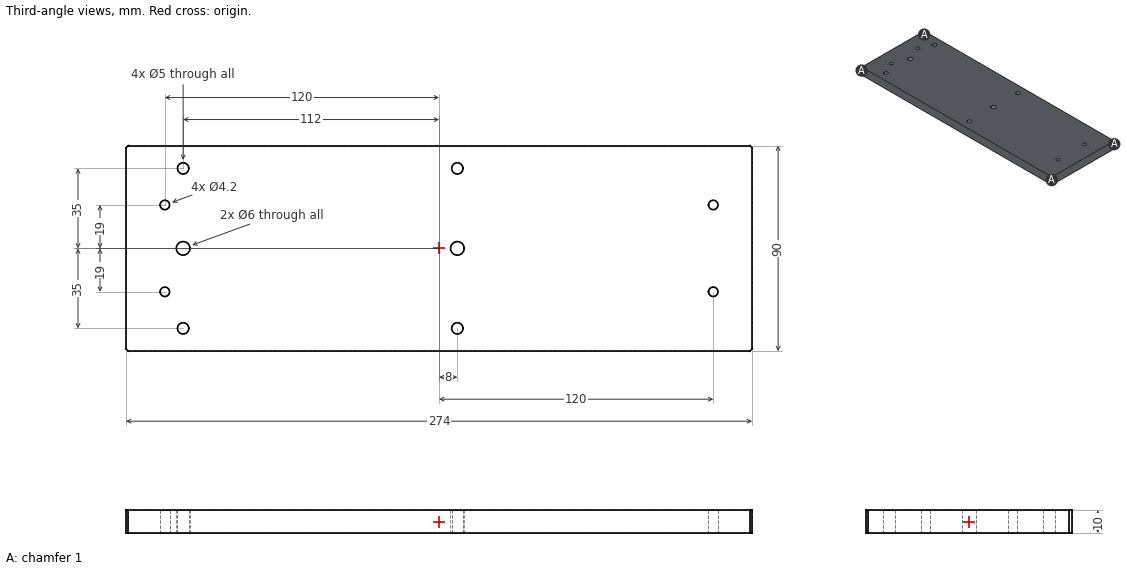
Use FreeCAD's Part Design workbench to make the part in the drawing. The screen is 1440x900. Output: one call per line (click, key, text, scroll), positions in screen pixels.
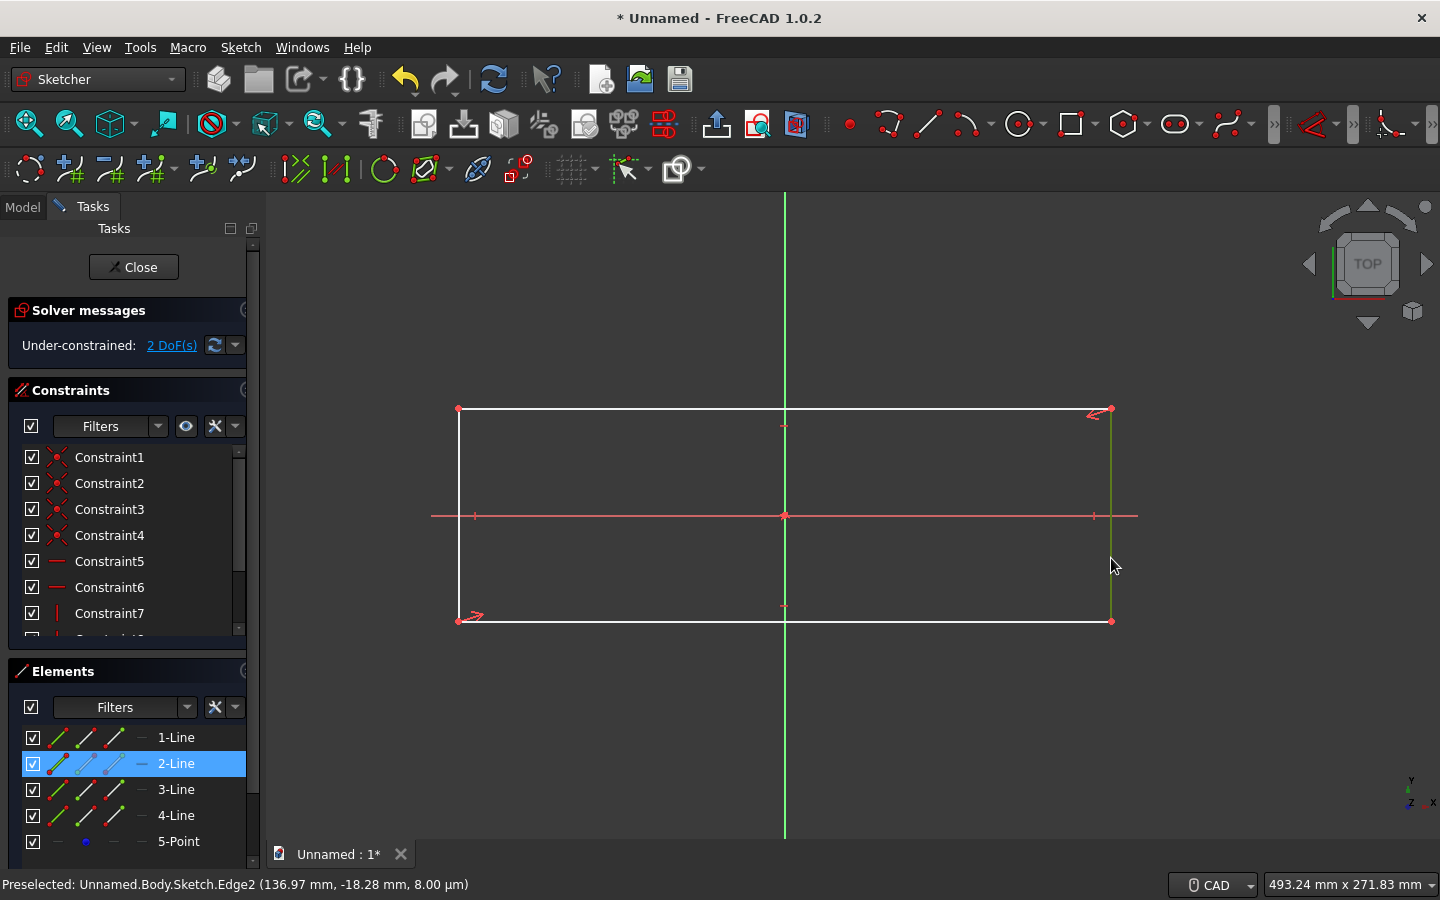
key(i)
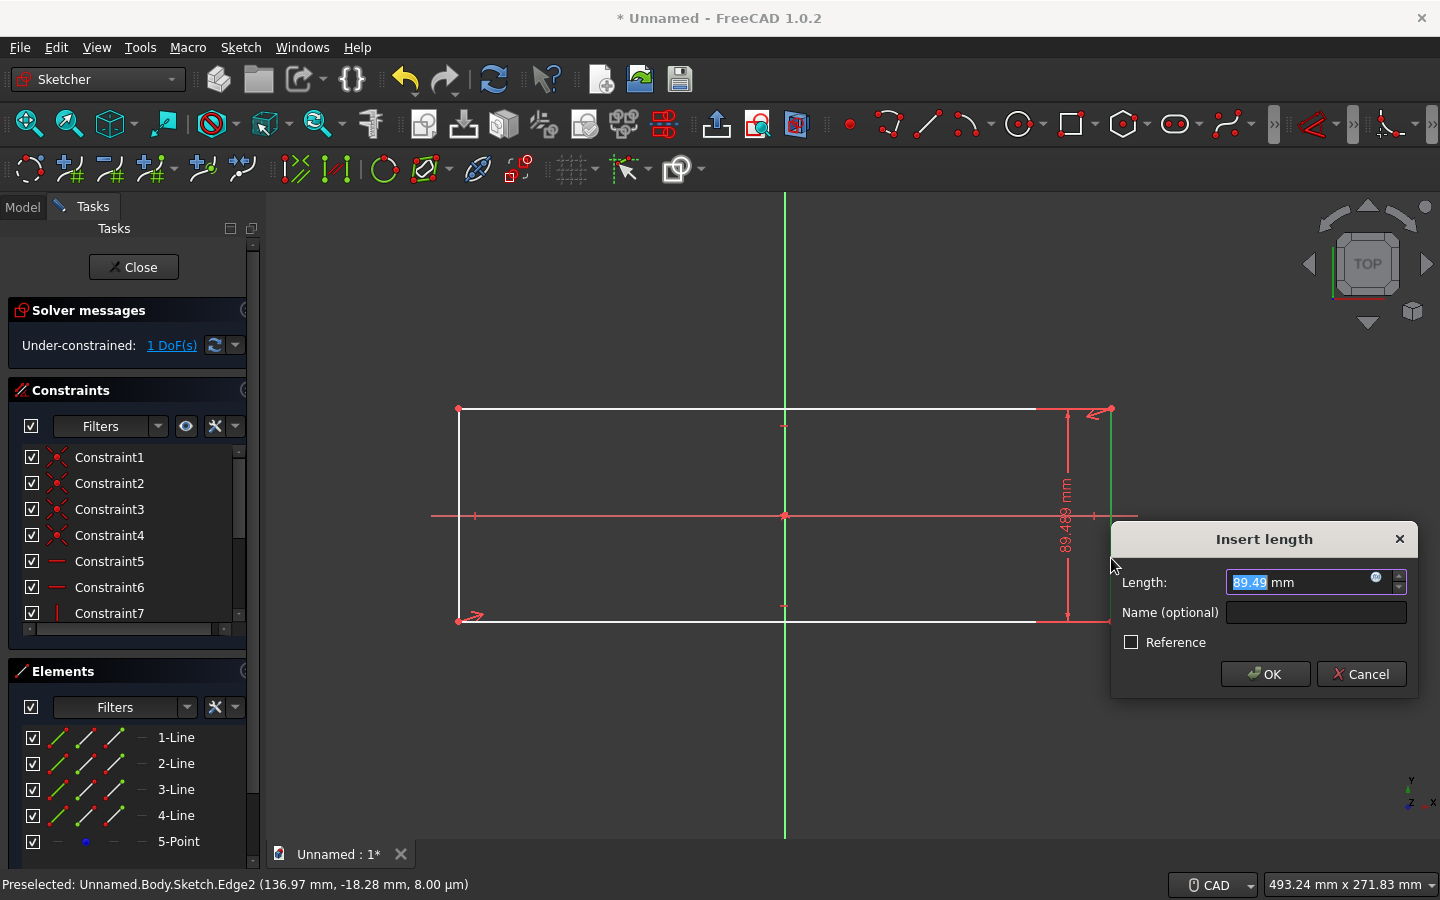
text(90)
key(Return)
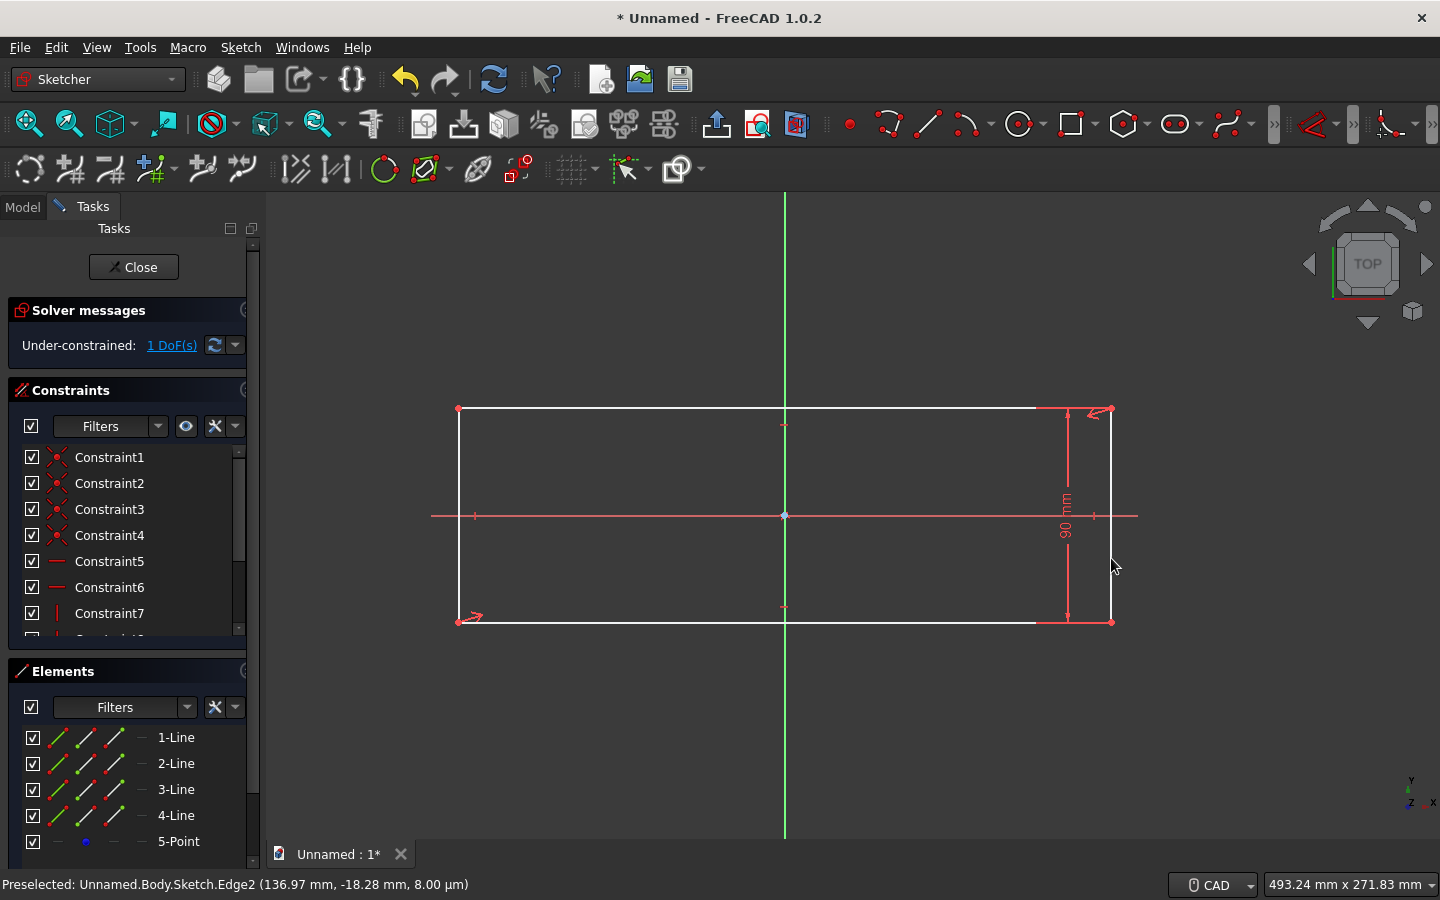
click(655, 623)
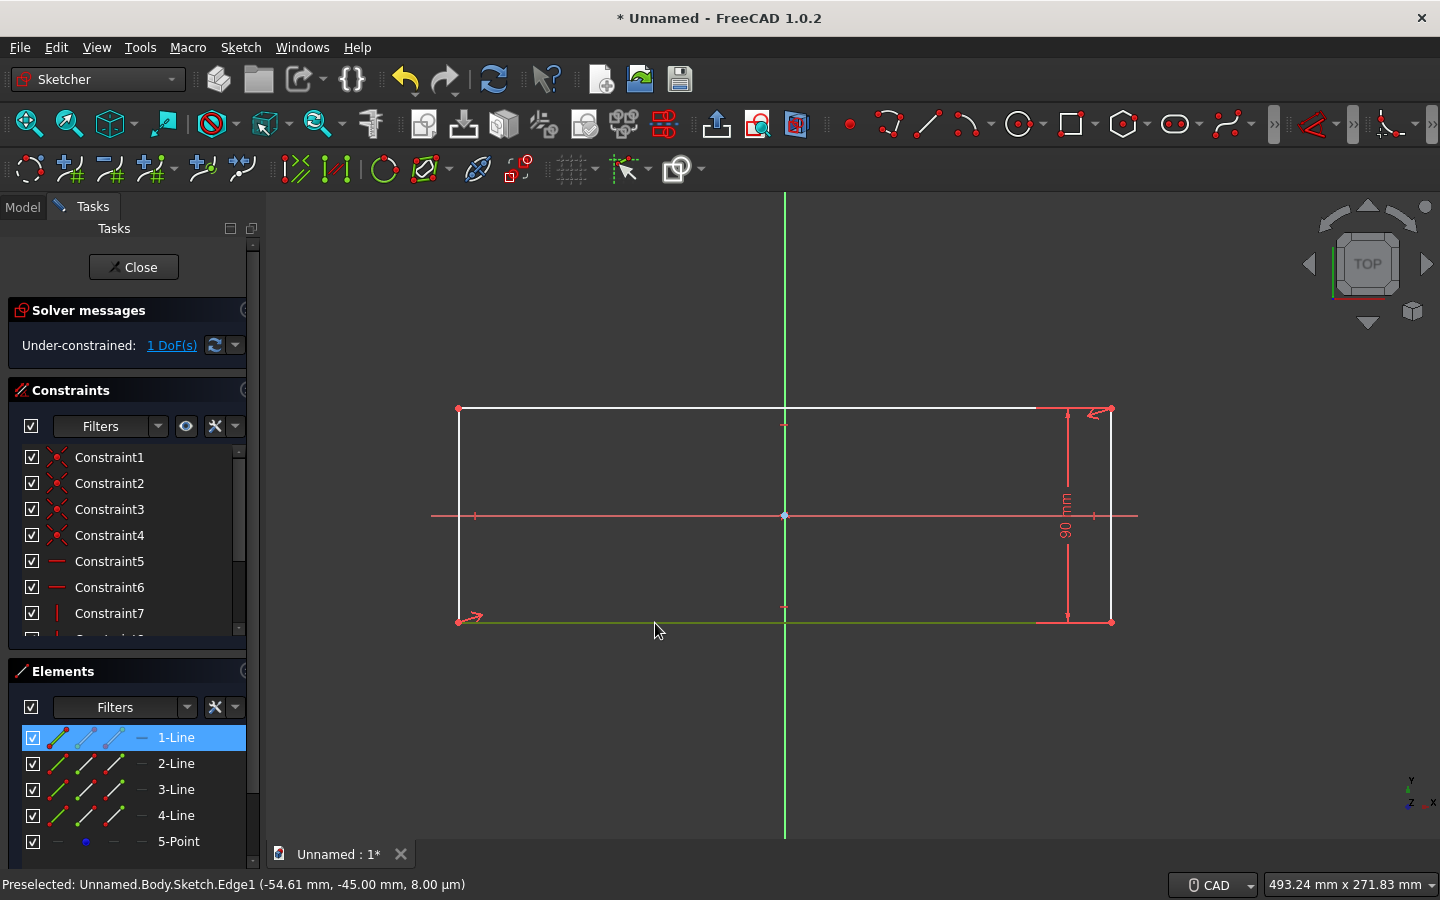
key(l)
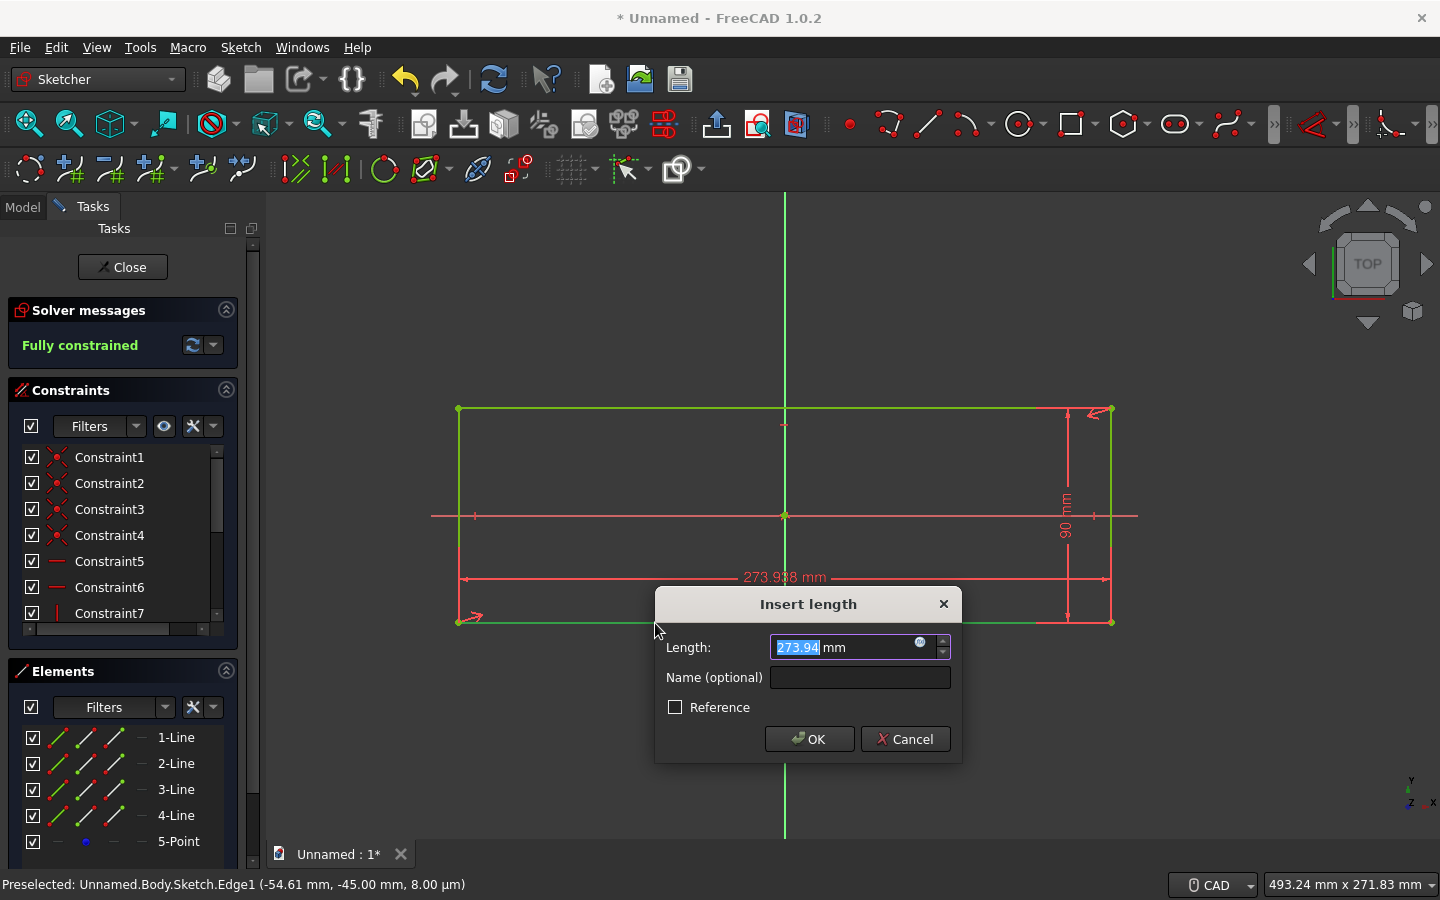
text(274)
key(Return)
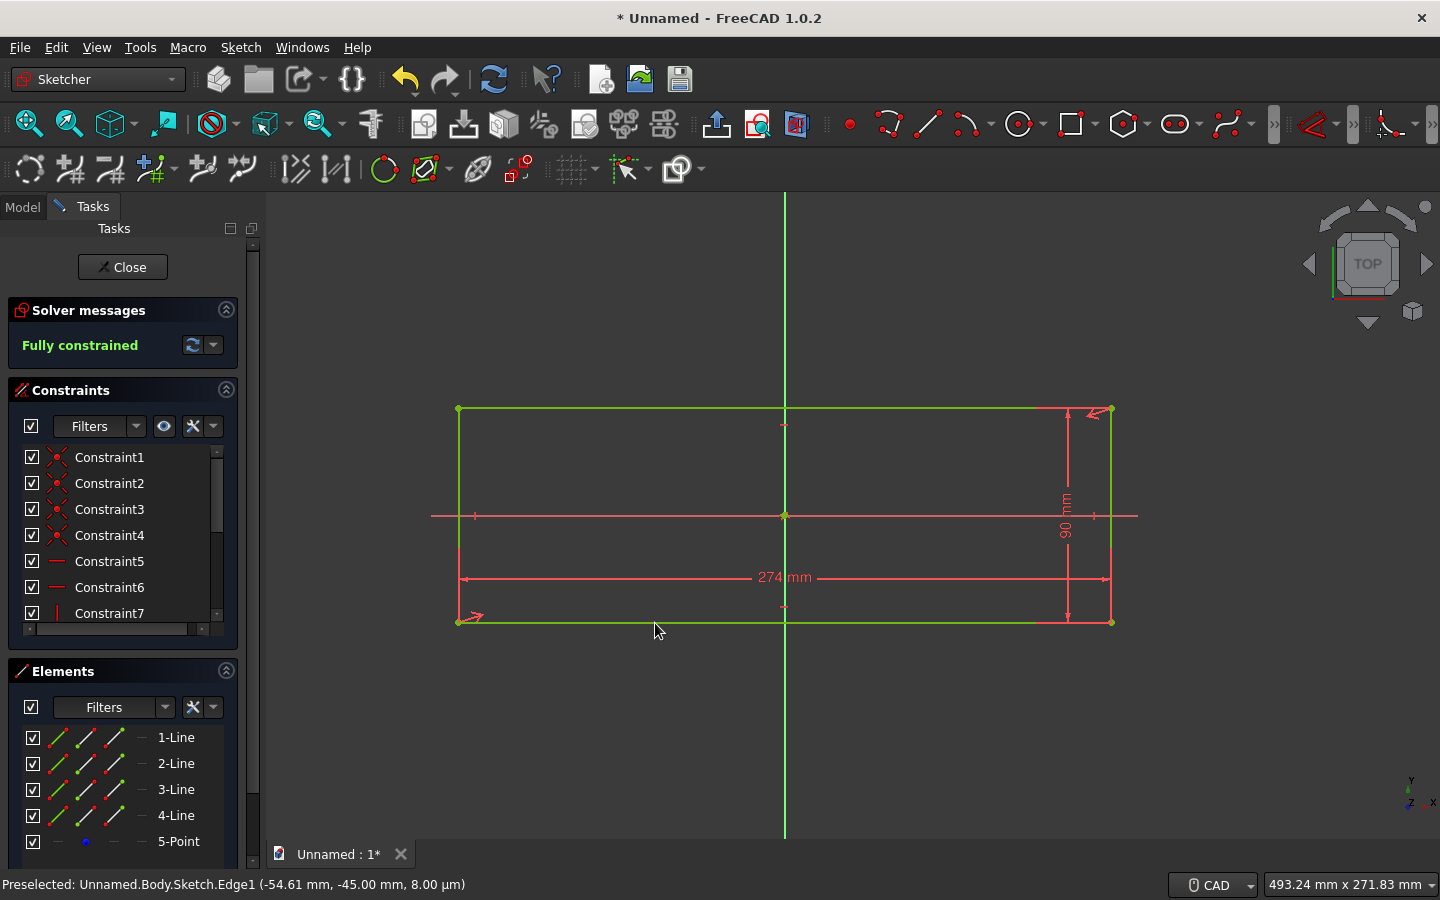
click(123, 267)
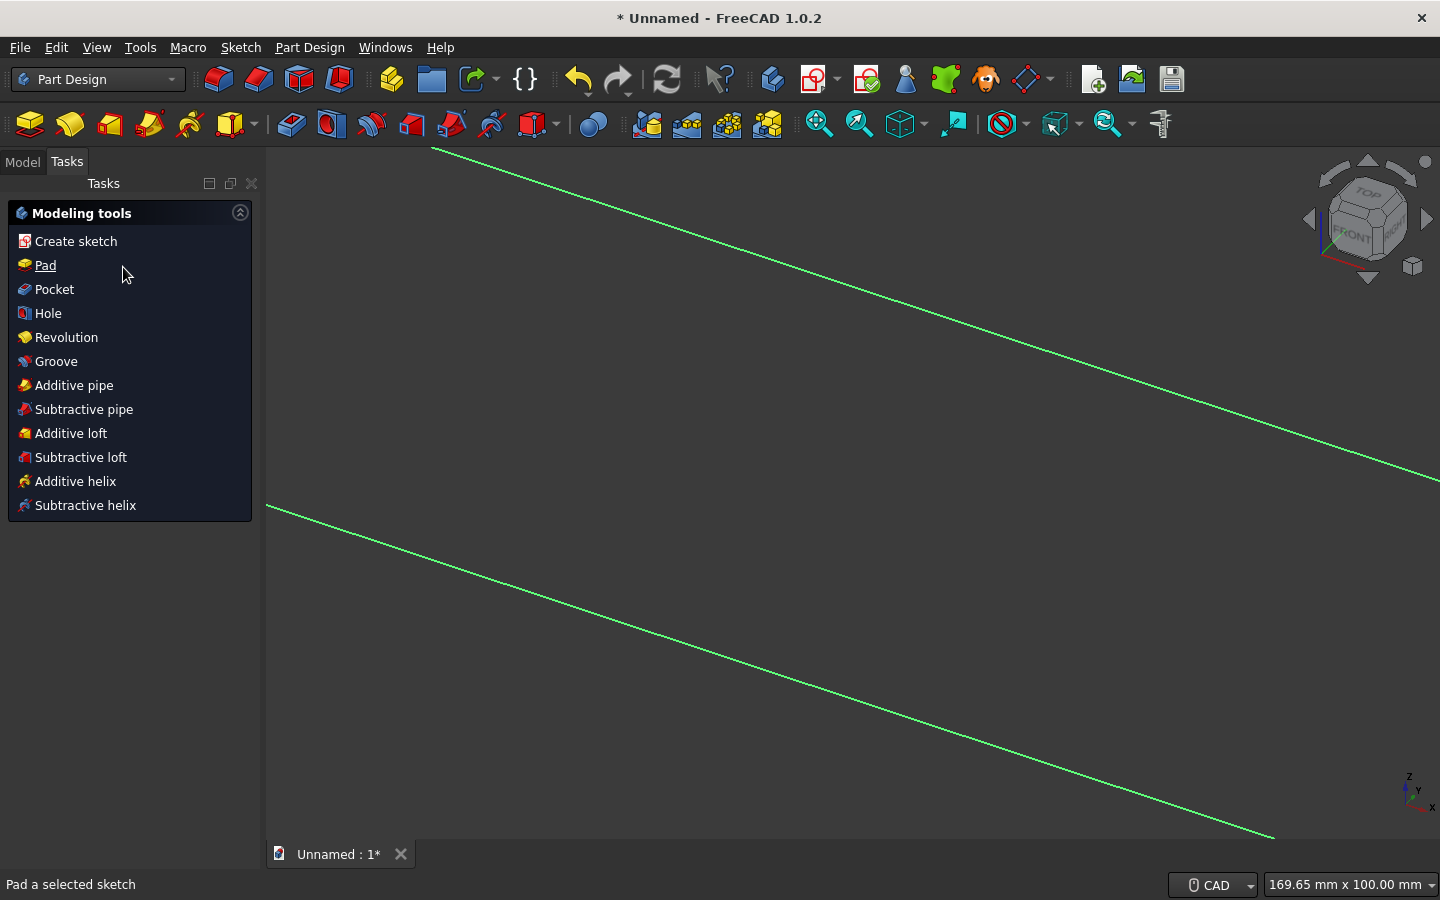
click(30, 124)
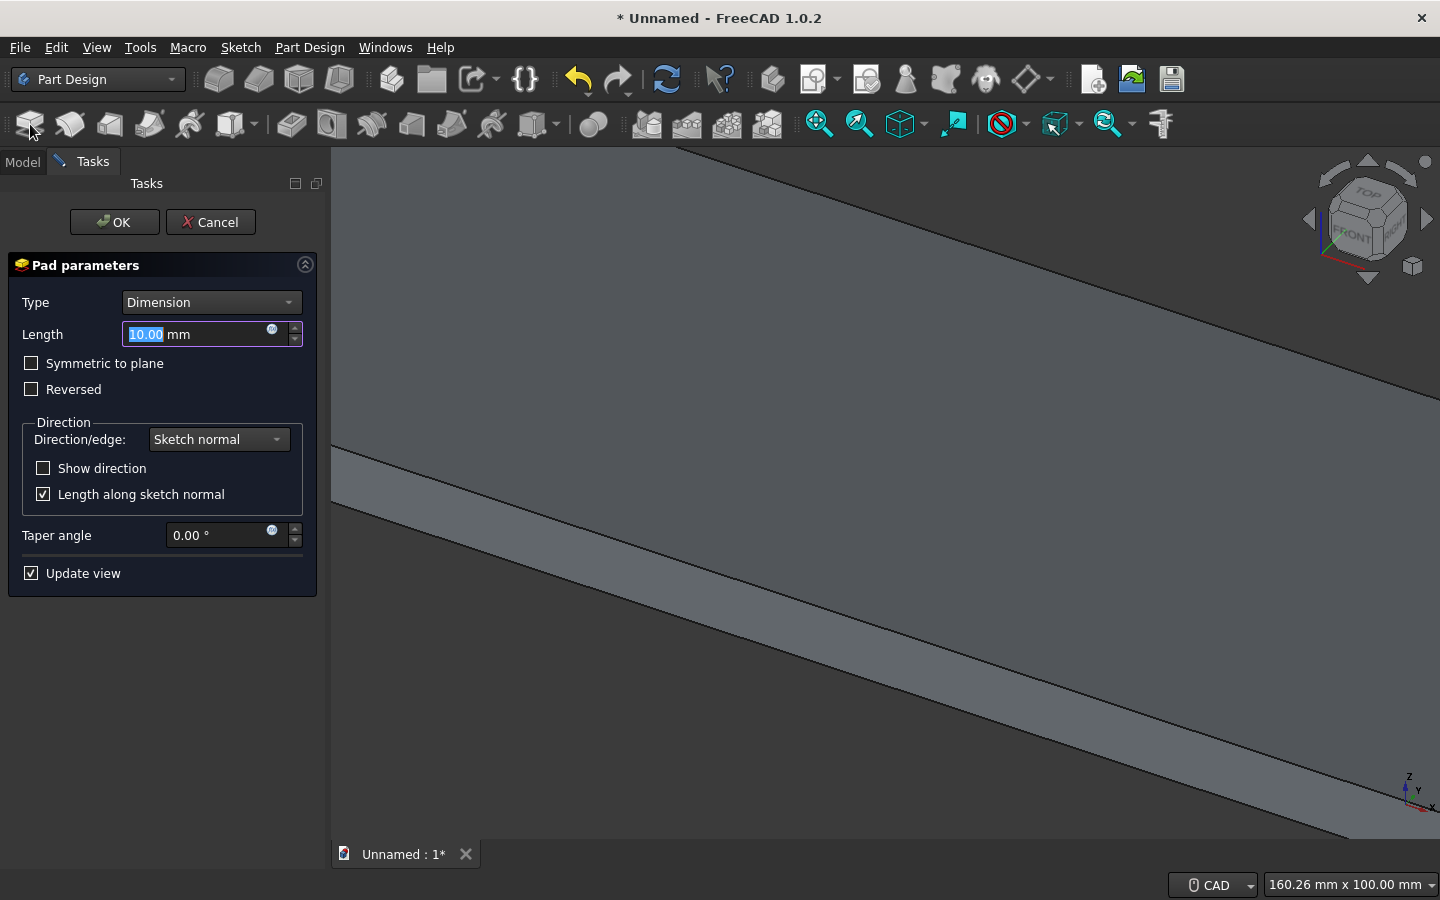
text(10)
key(Tab)